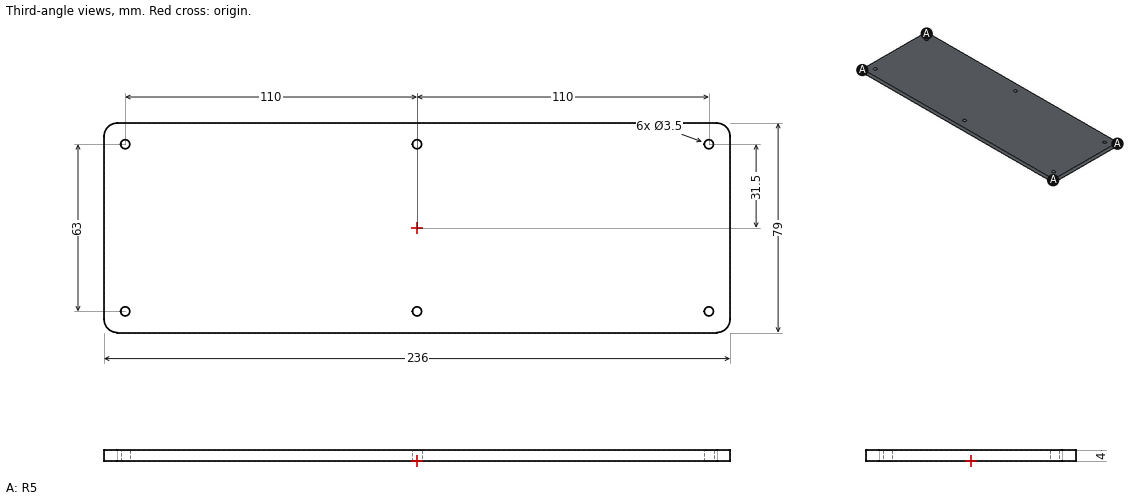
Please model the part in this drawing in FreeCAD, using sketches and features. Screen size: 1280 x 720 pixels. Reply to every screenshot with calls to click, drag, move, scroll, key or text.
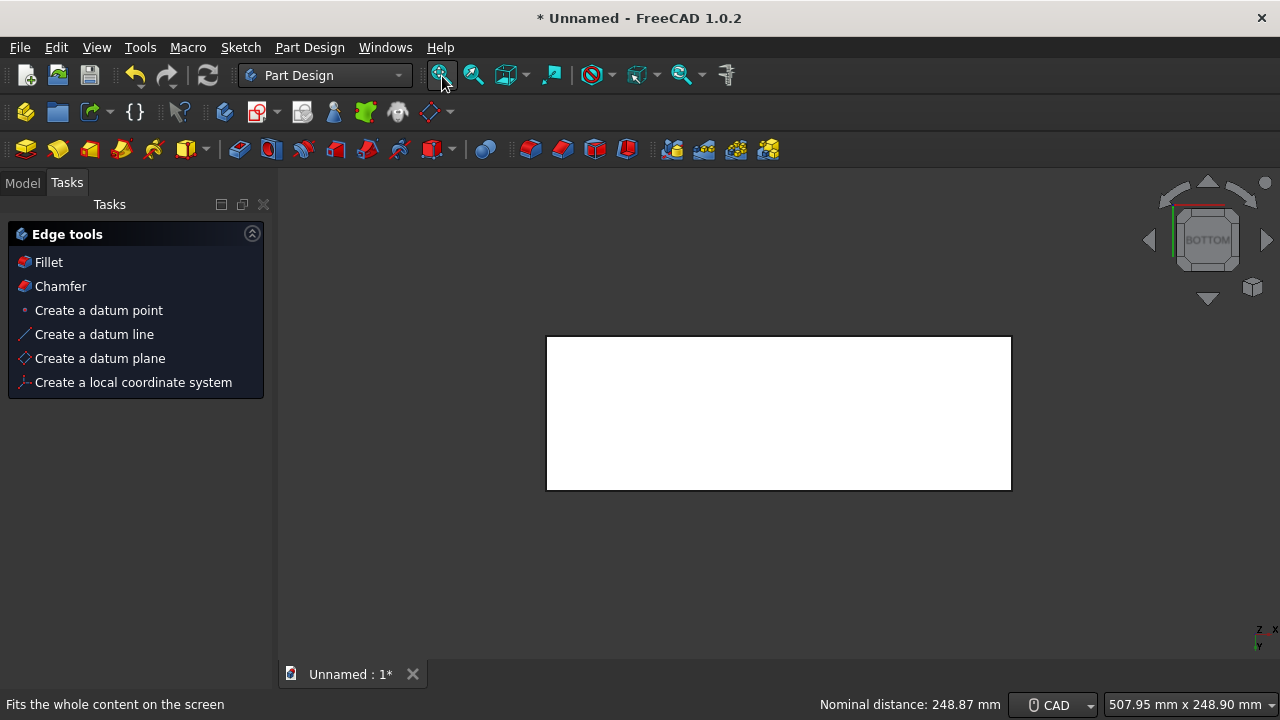
key(4)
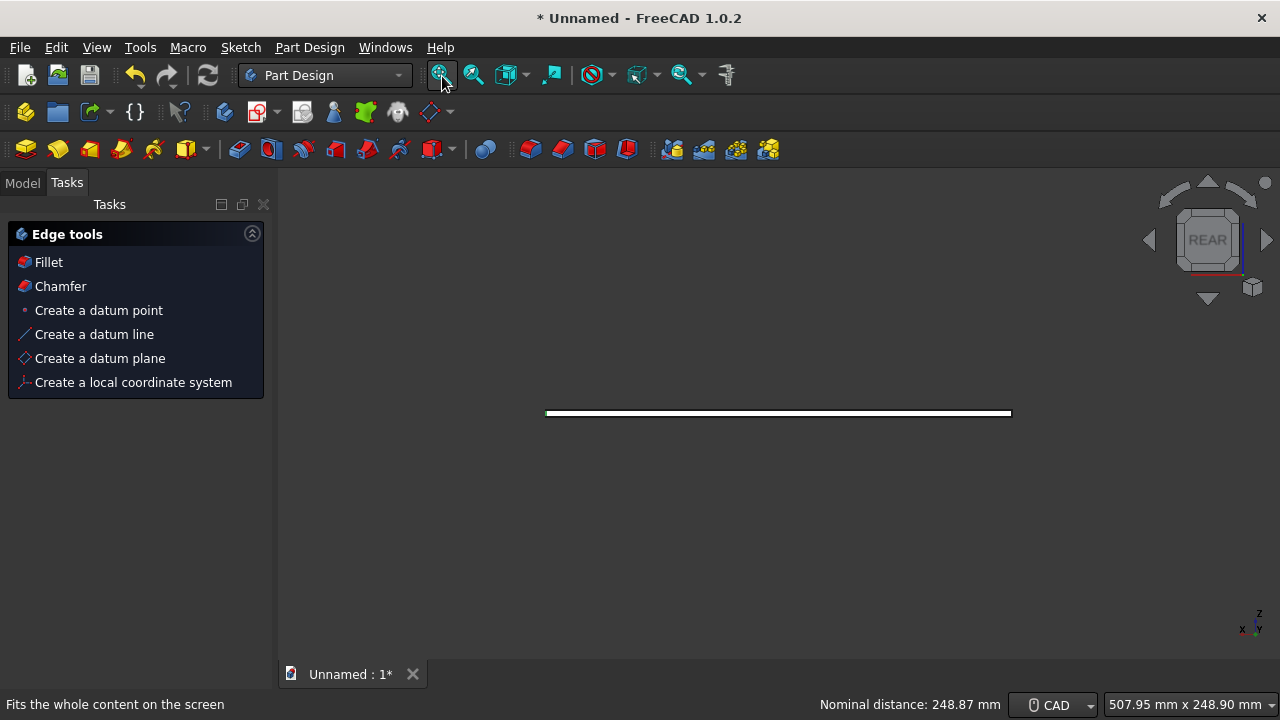
scroll(1012, 412, up, 9)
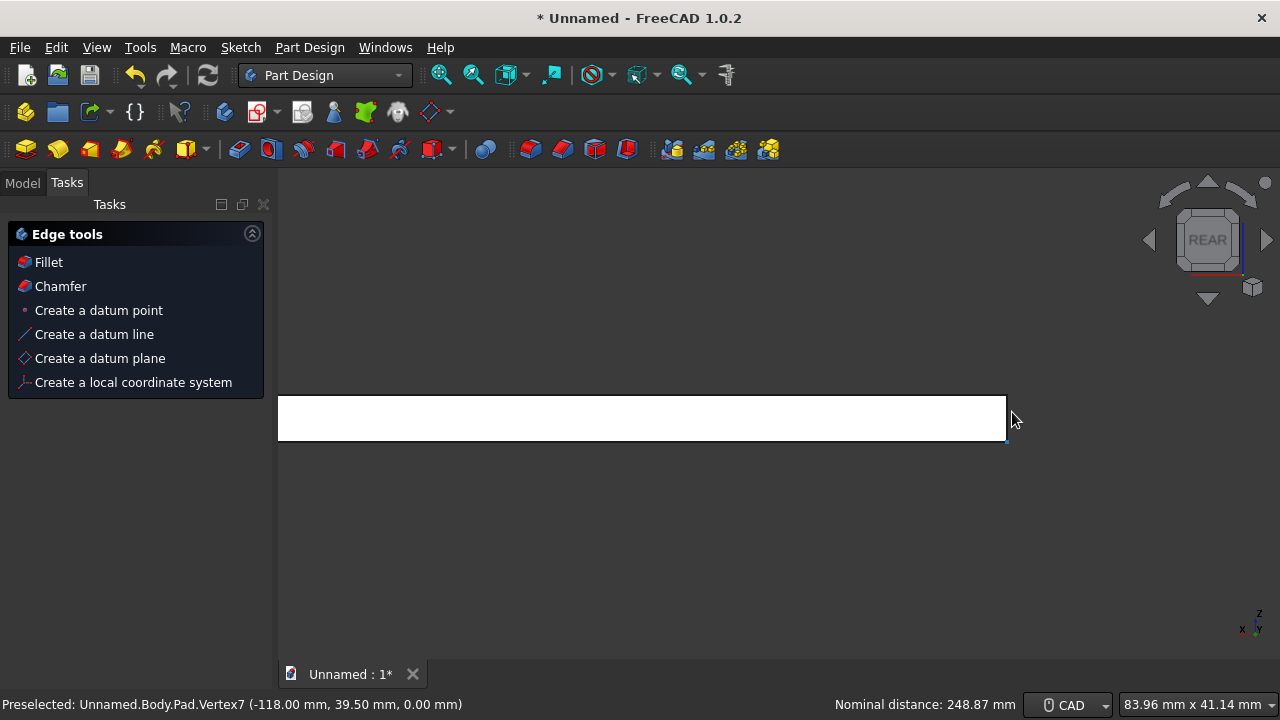
click(1007, 418, ctrl)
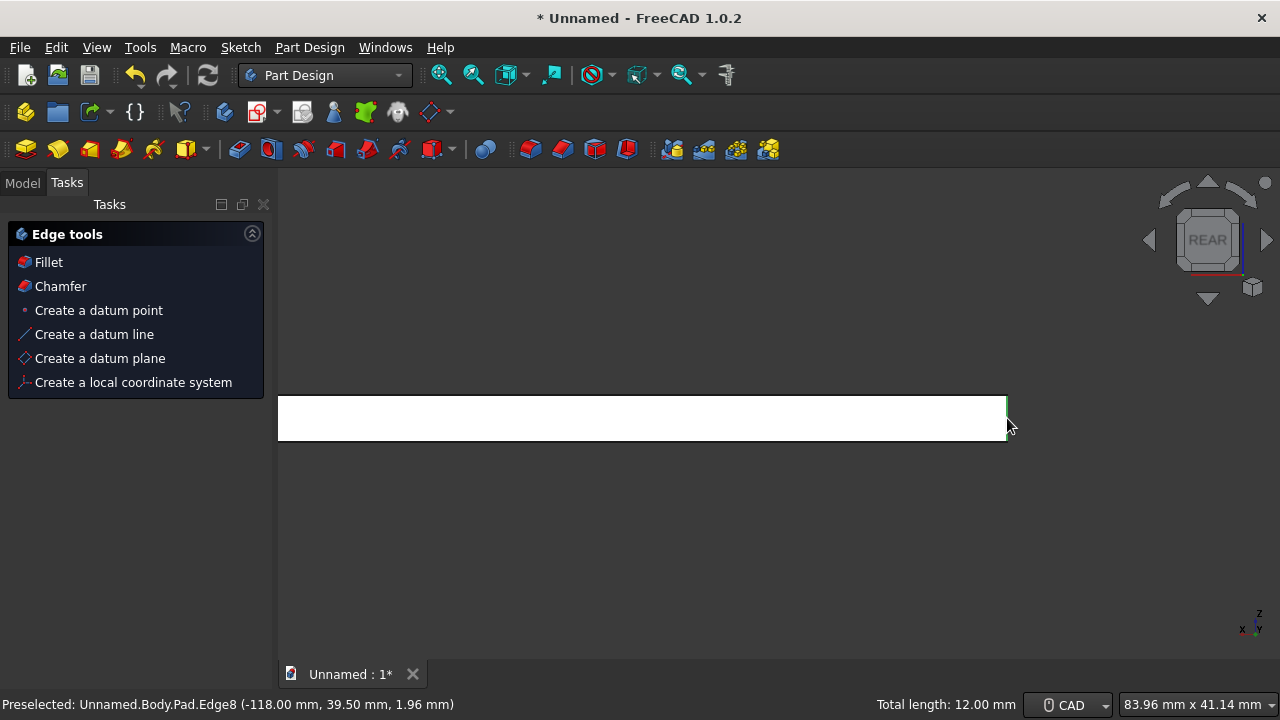
click(442, 76)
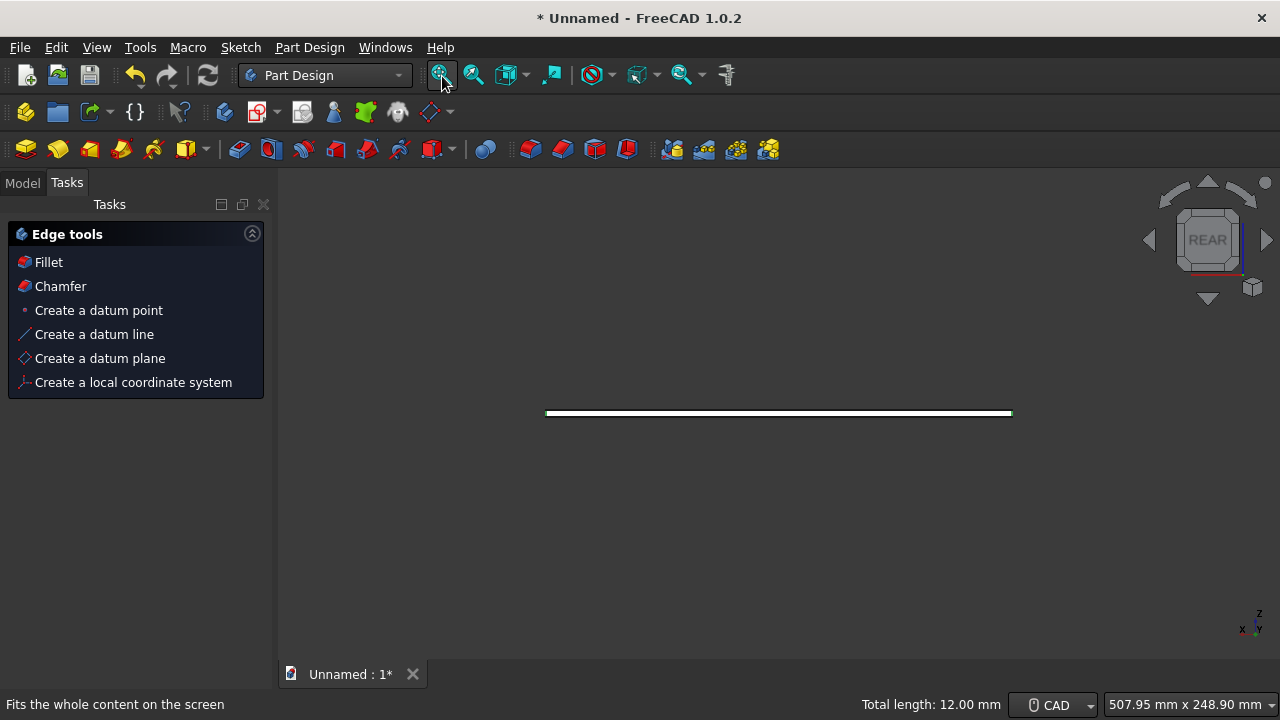
key(6)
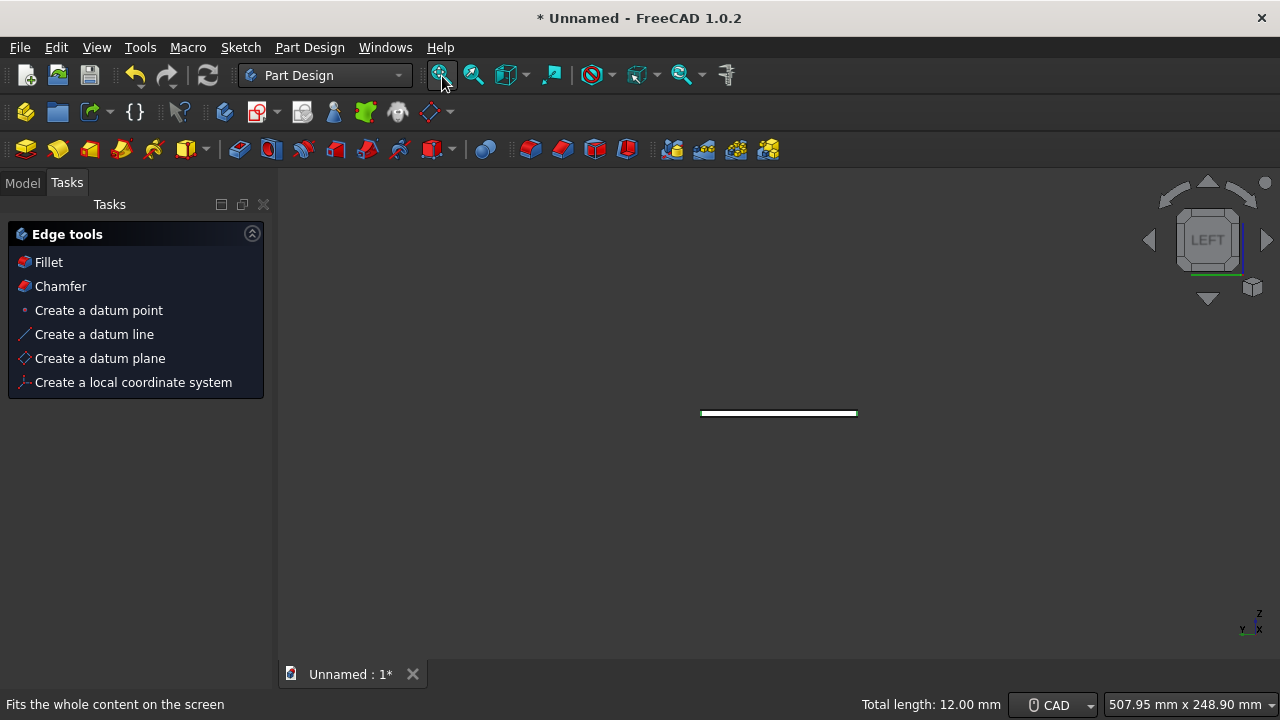
click(442, 76)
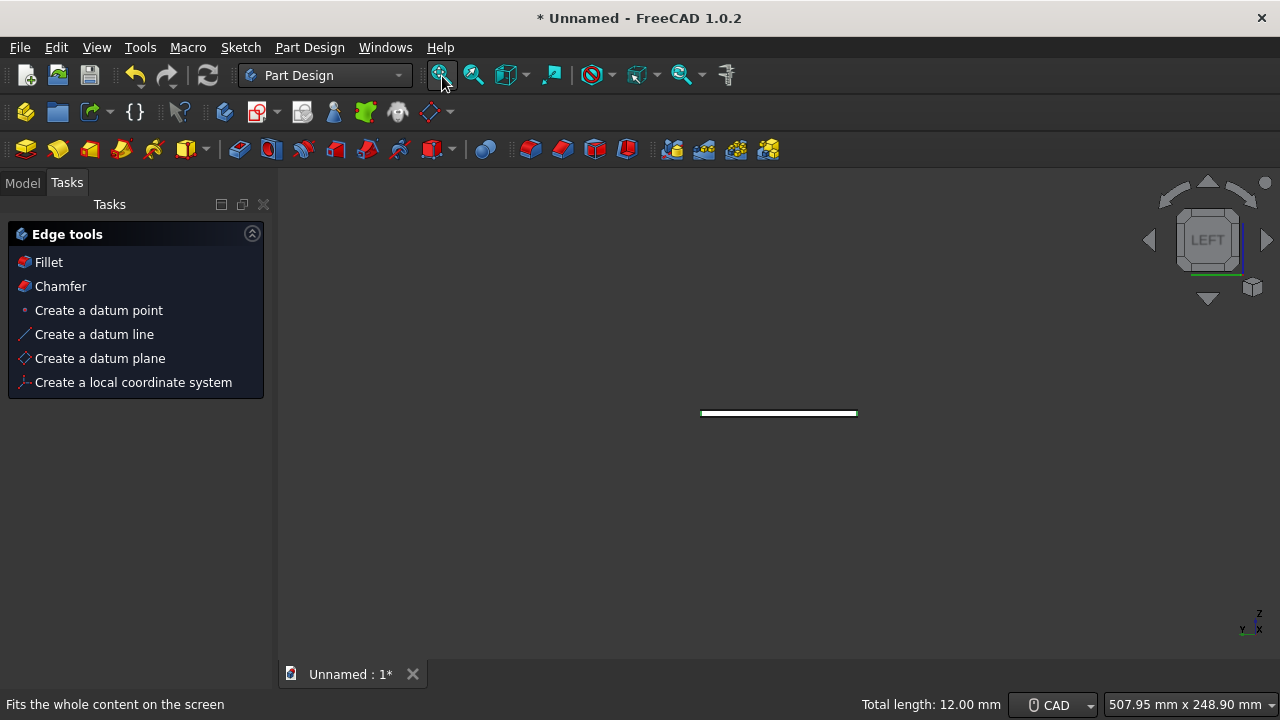
scroll(857, 412, up, 9)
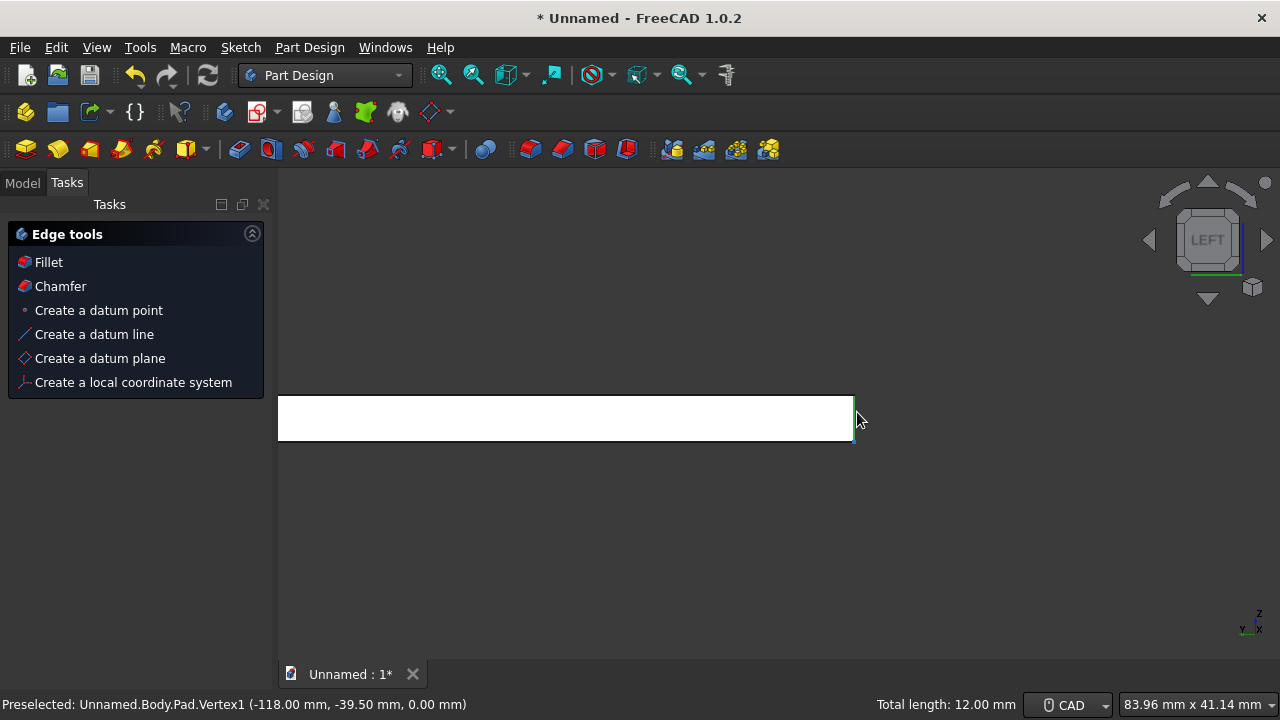
click(442, 76)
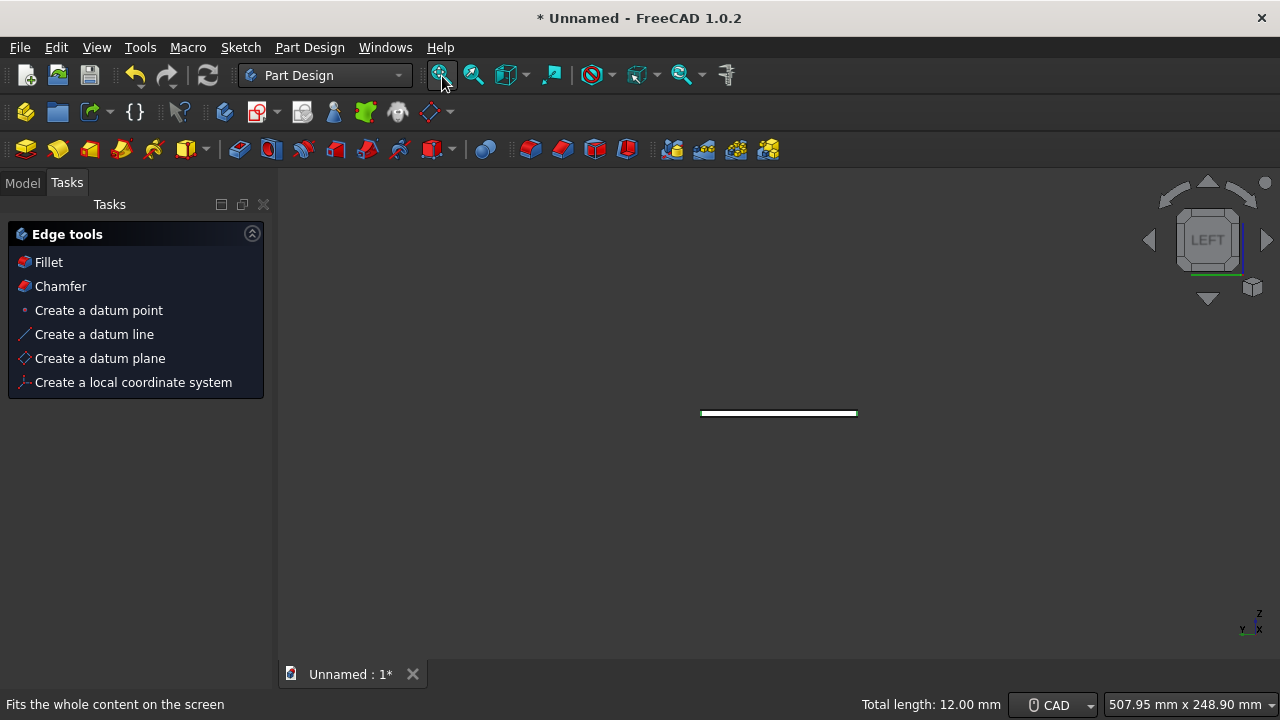
key(v)
key(3)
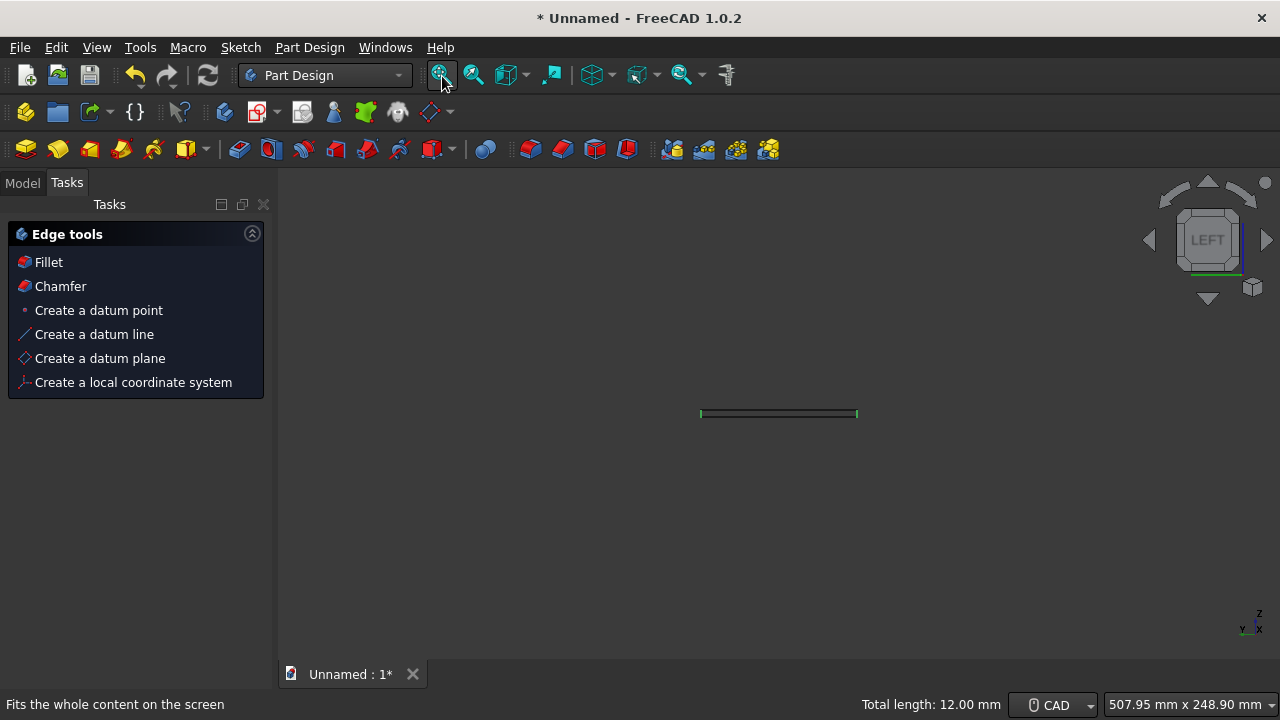
key(0)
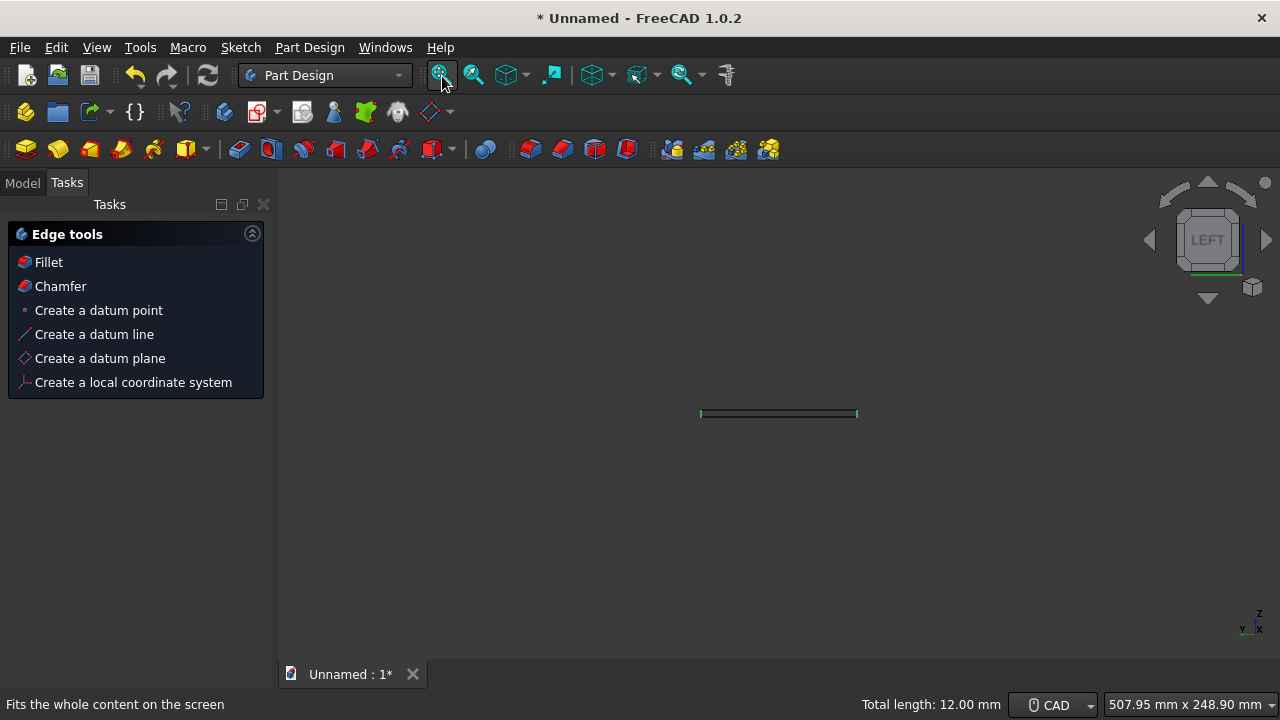
scroll(888, 539, up, 9)